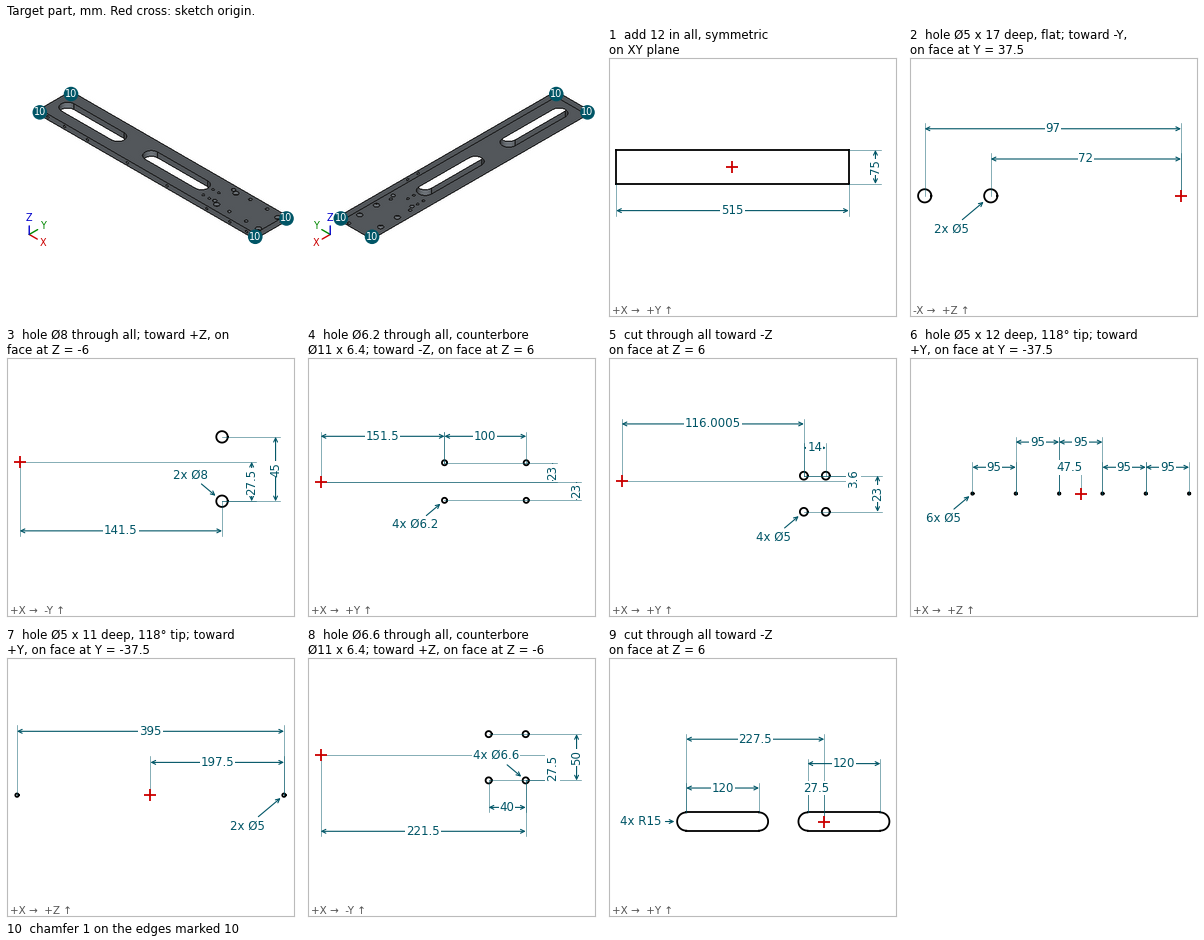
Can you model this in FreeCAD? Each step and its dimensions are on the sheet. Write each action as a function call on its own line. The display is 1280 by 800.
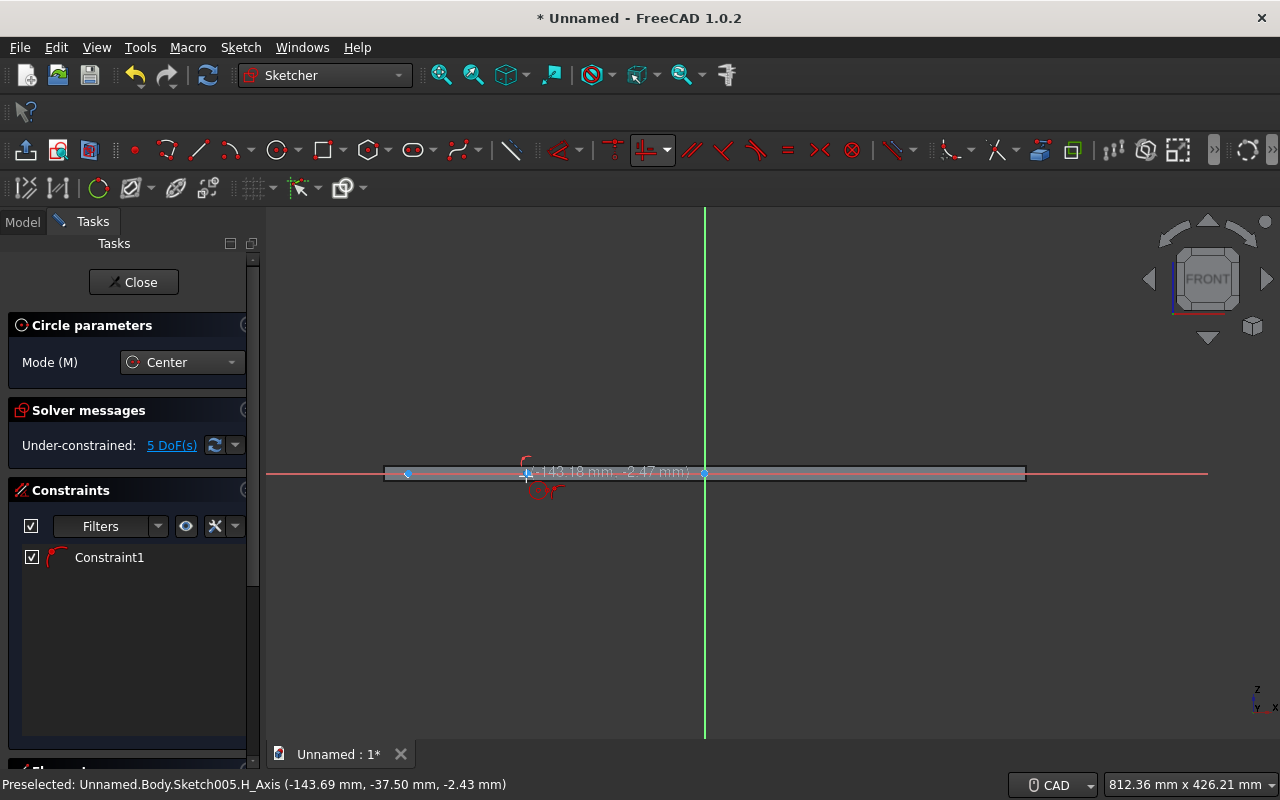
scroll(646, 473, up, 10)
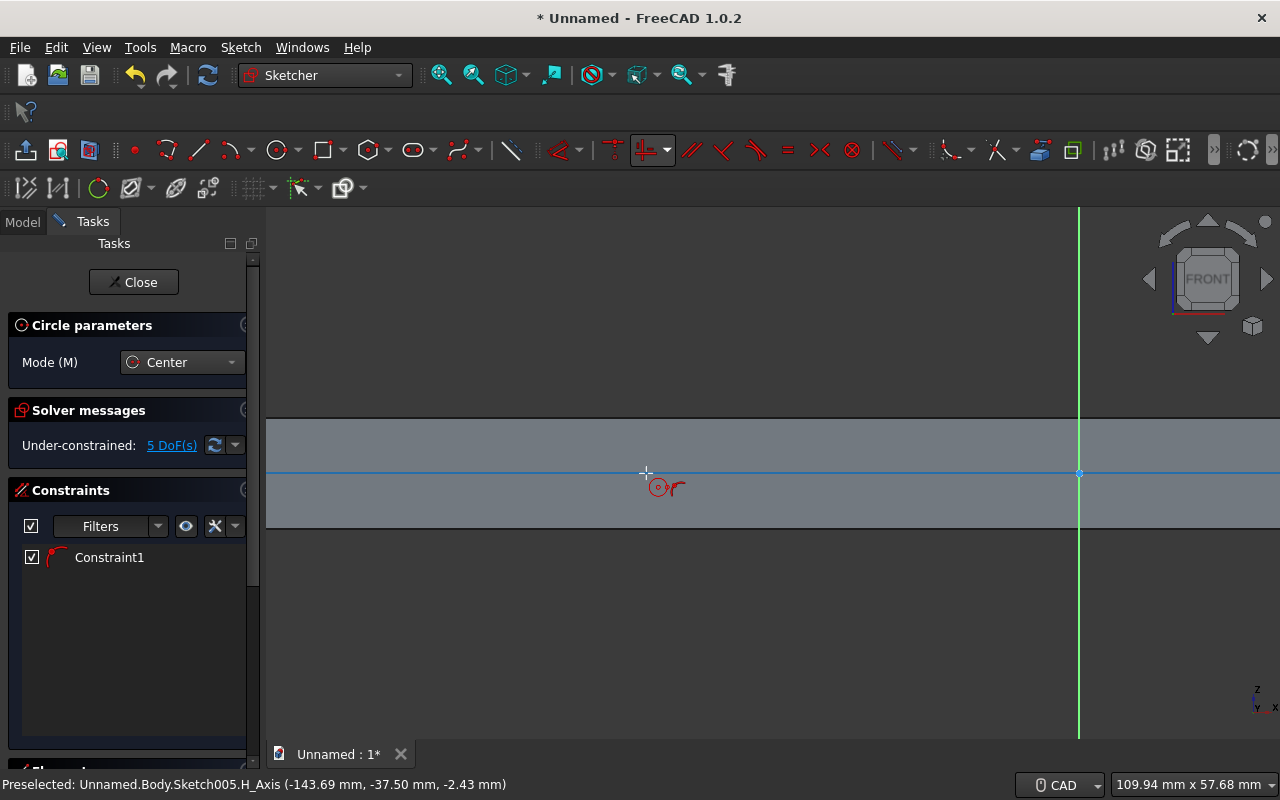
scroll(646, 473, down, 10)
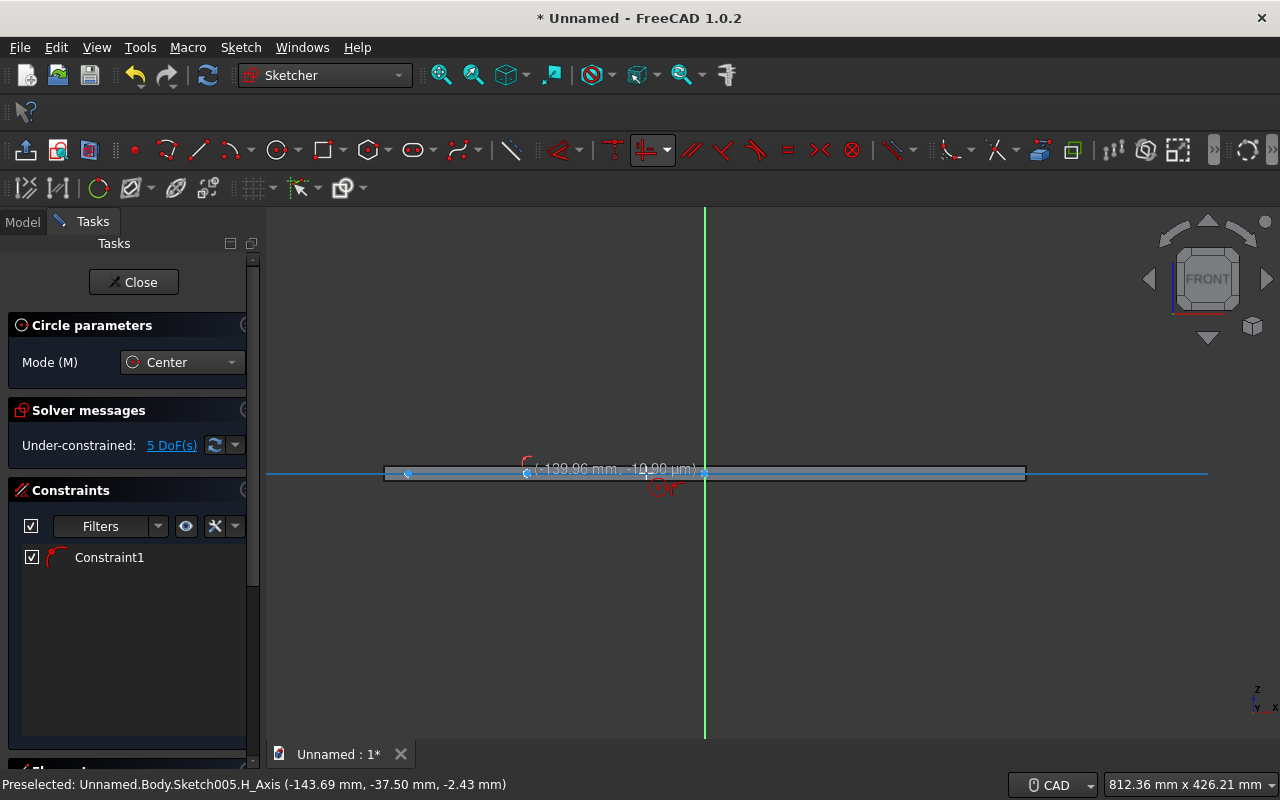
click(646, 473)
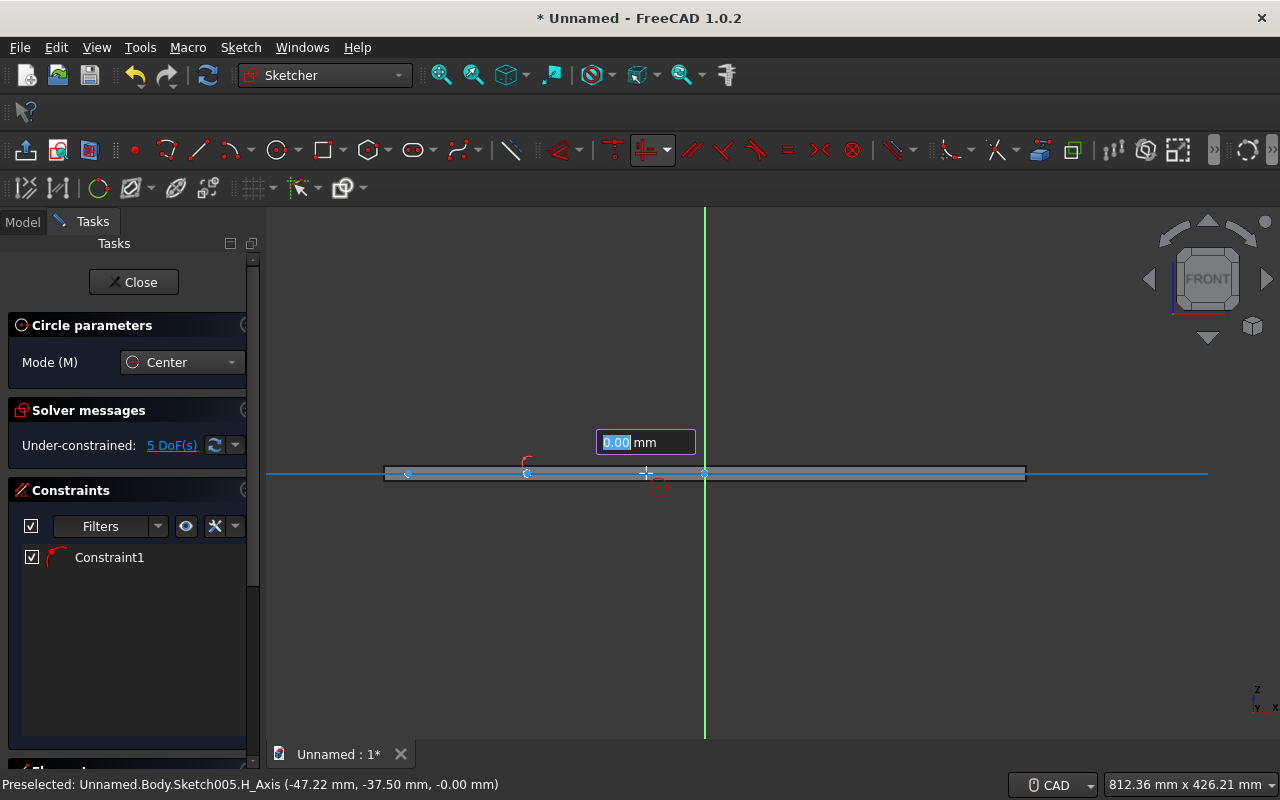
scroll(645, 476, up, 9)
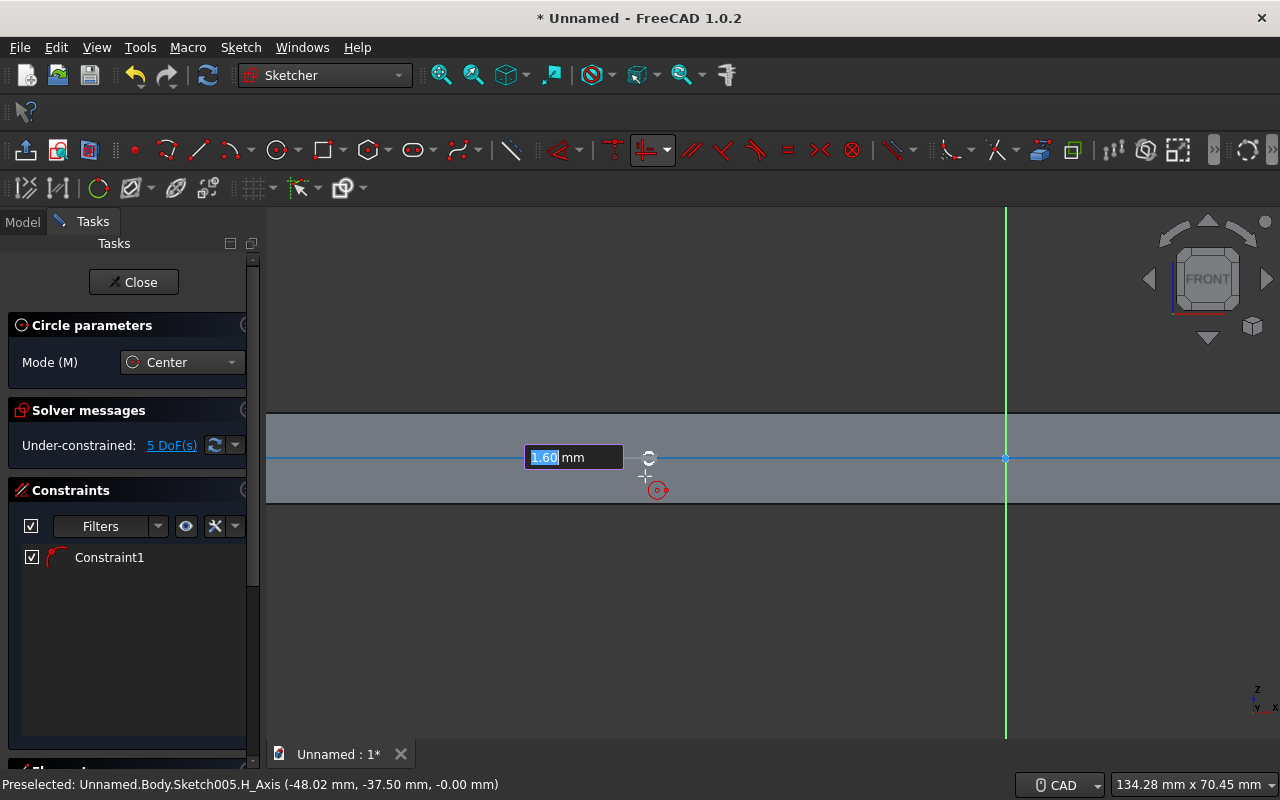
click(641, 476)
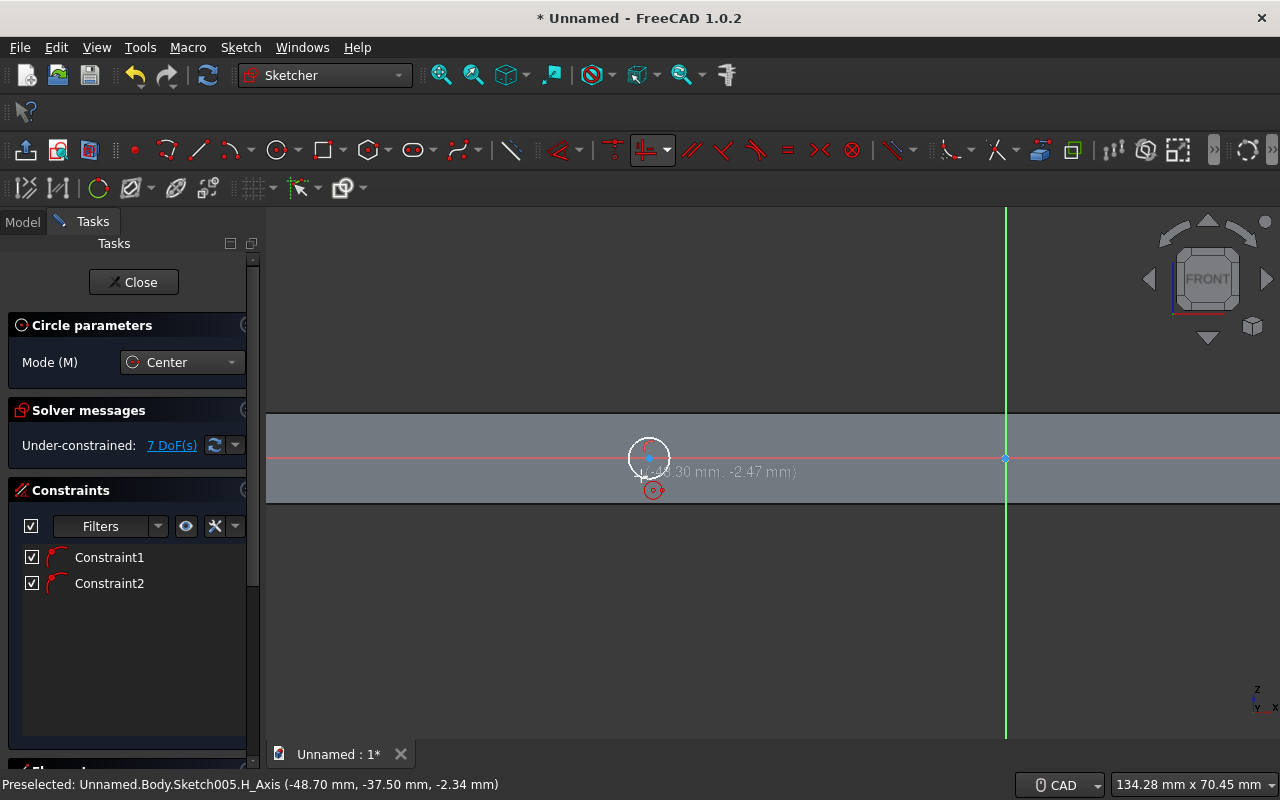
scroll(645, 476, down, 9)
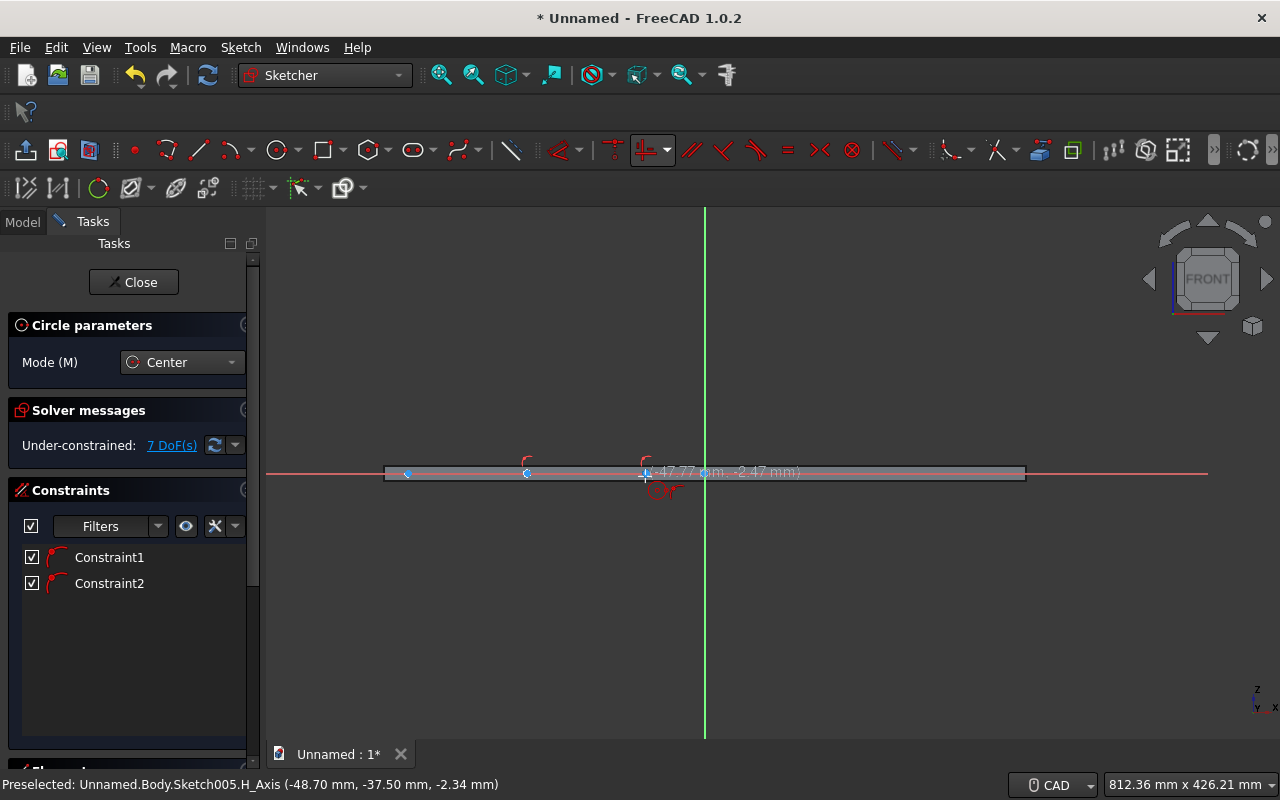
scroll(764, 473, up, 10)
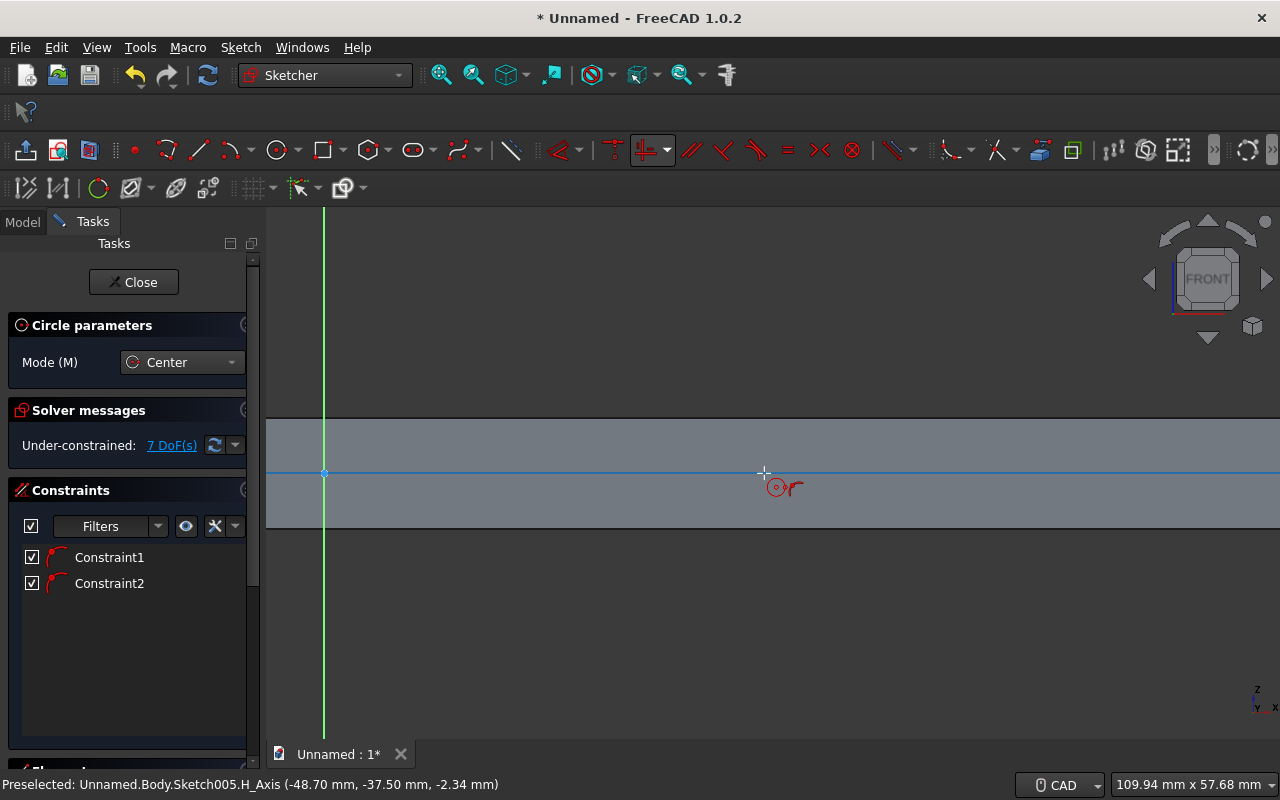
scroll(764, 473, down, 10)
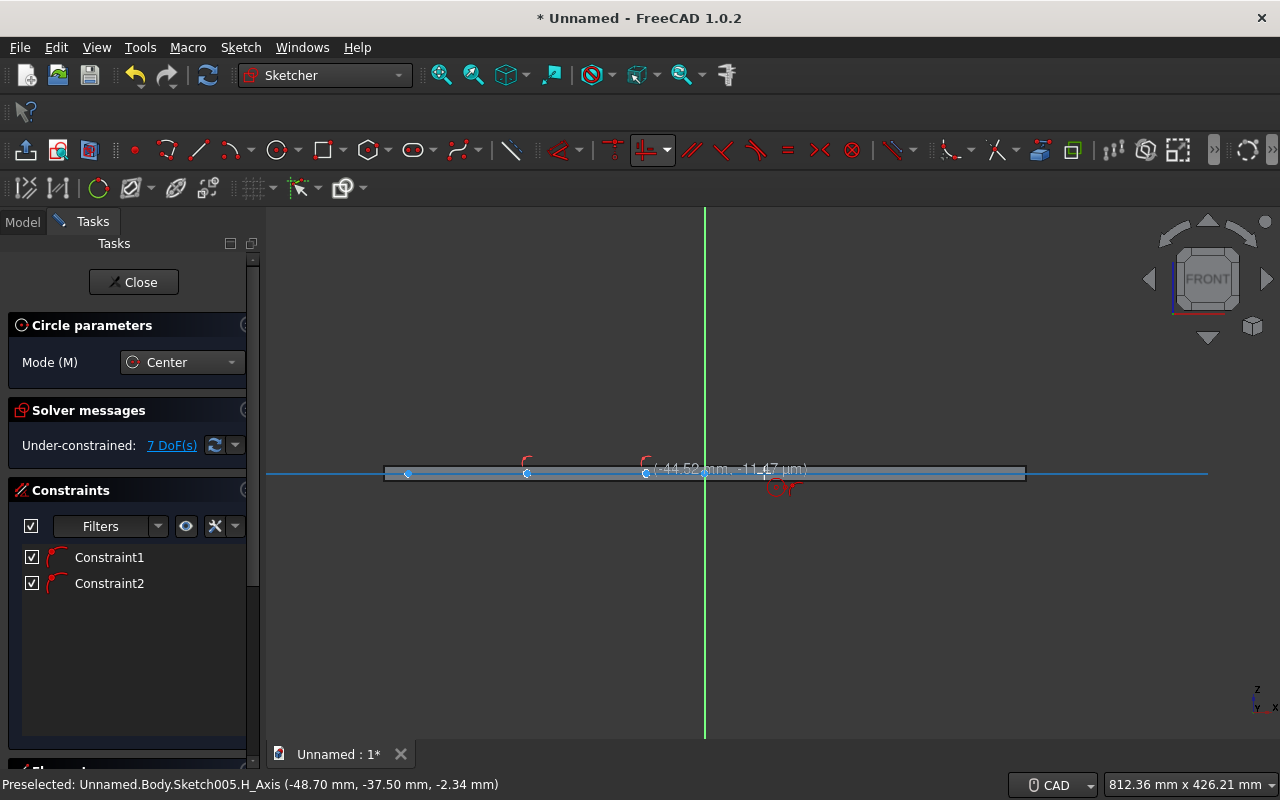
click(764, 473)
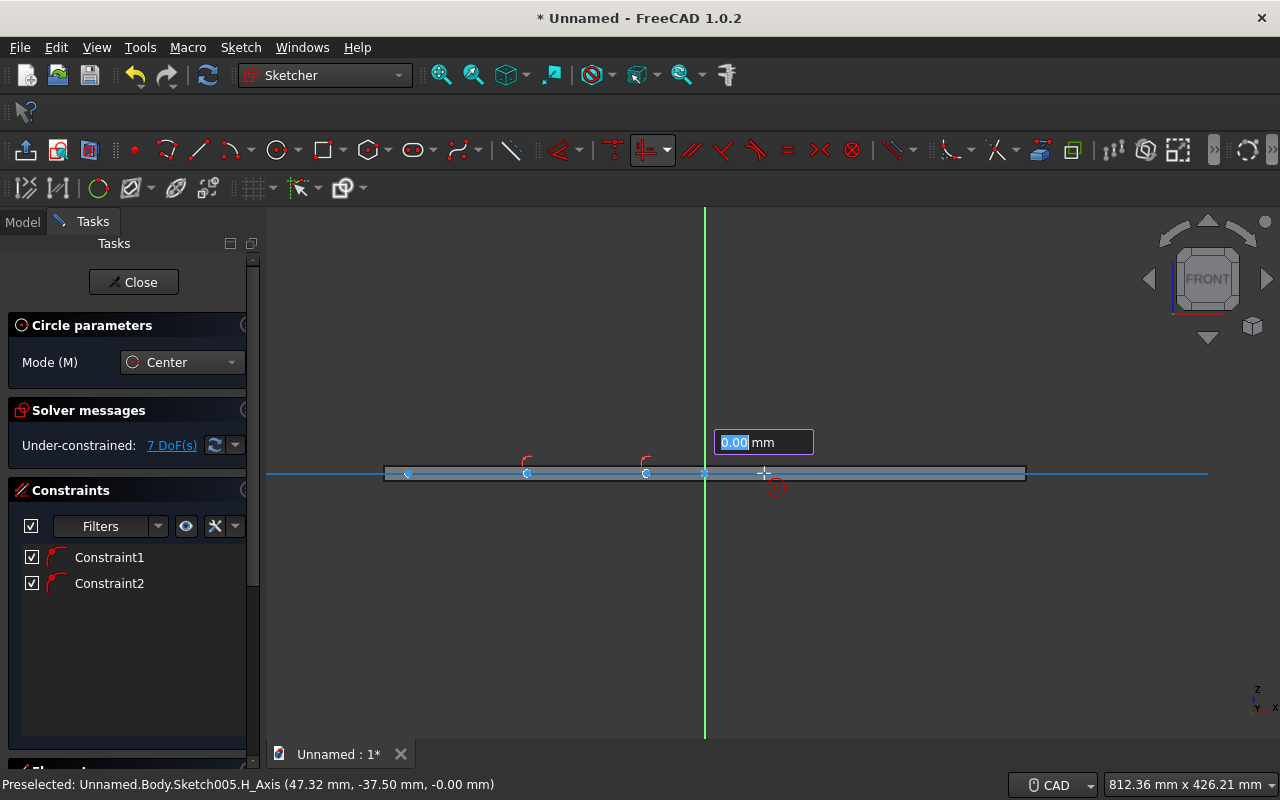
scroll(763, 476, up, 9)